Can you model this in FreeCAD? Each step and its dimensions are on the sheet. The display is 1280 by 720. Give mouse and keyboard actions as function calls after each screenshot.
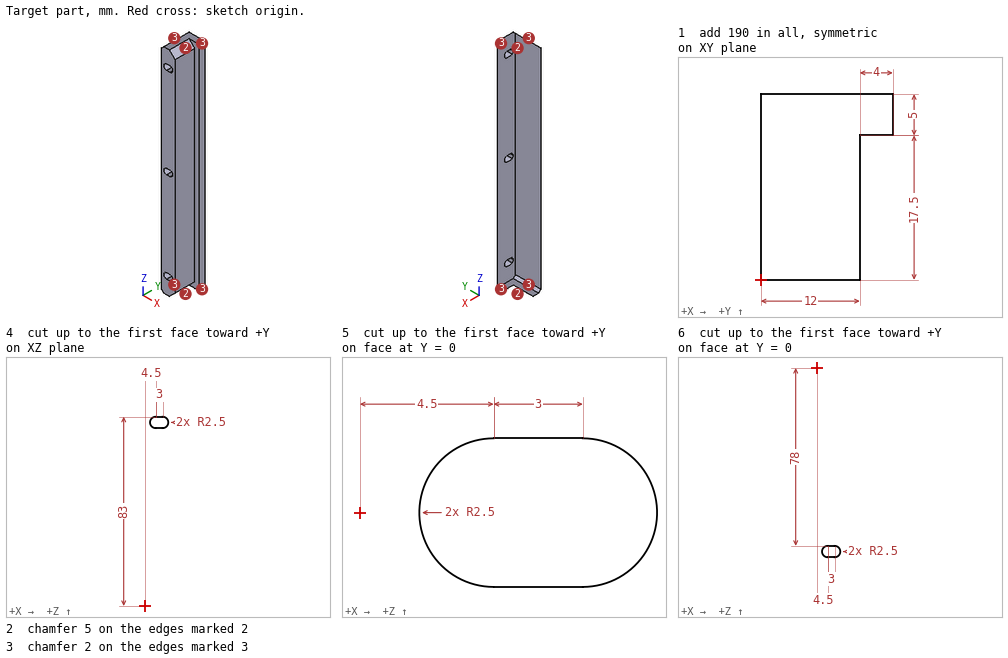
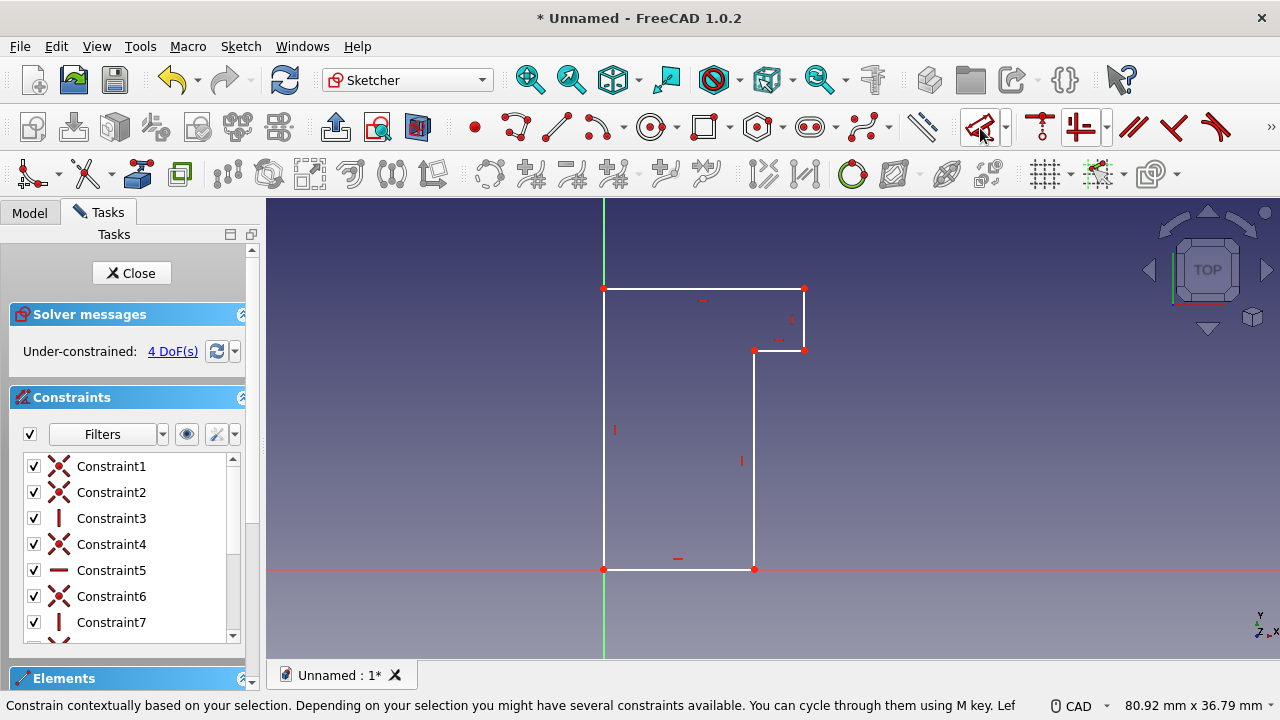
click(769, 351)
click(779, 317)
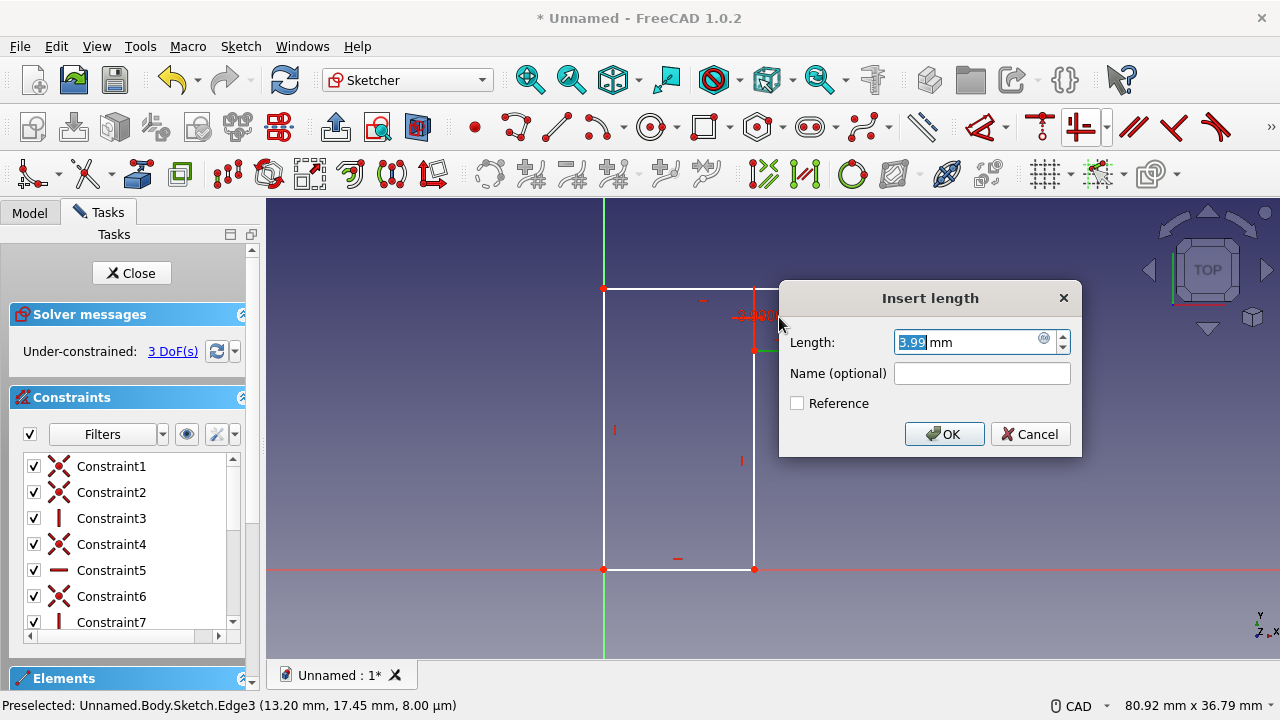
text(4)
key(Return)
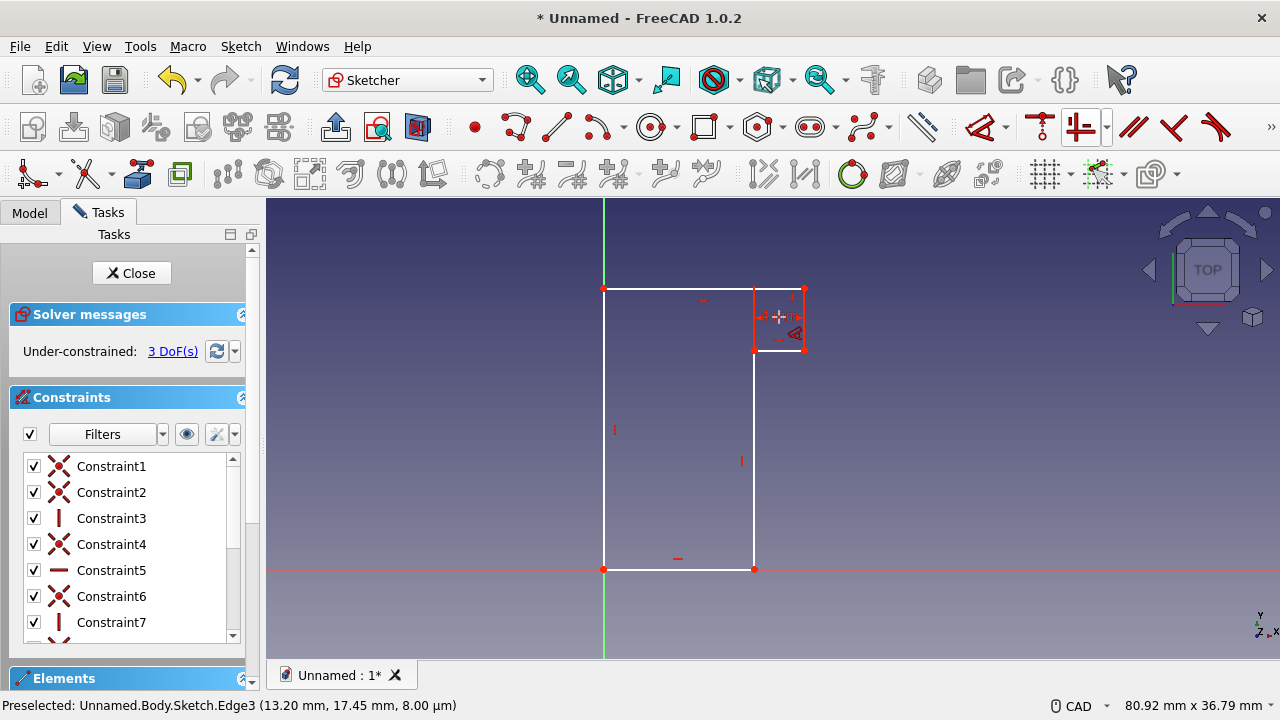
click(804, 332)
click(838, 342)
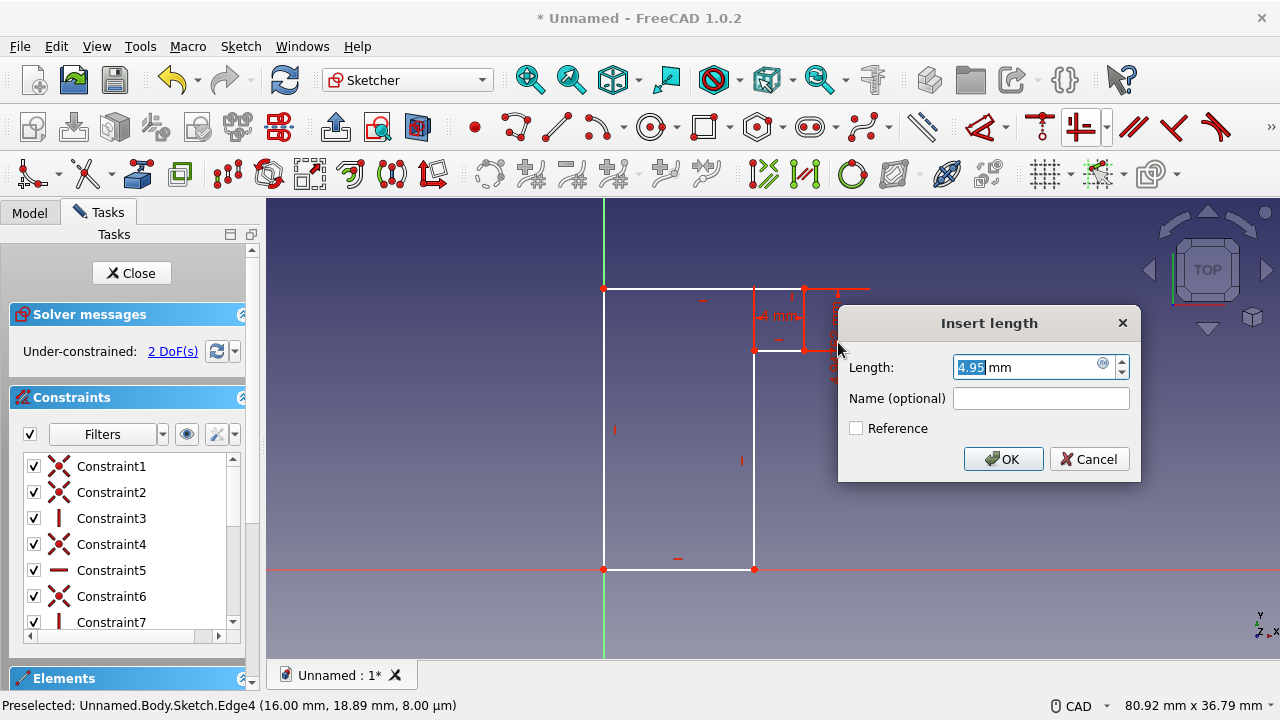
text(5)
key(Return)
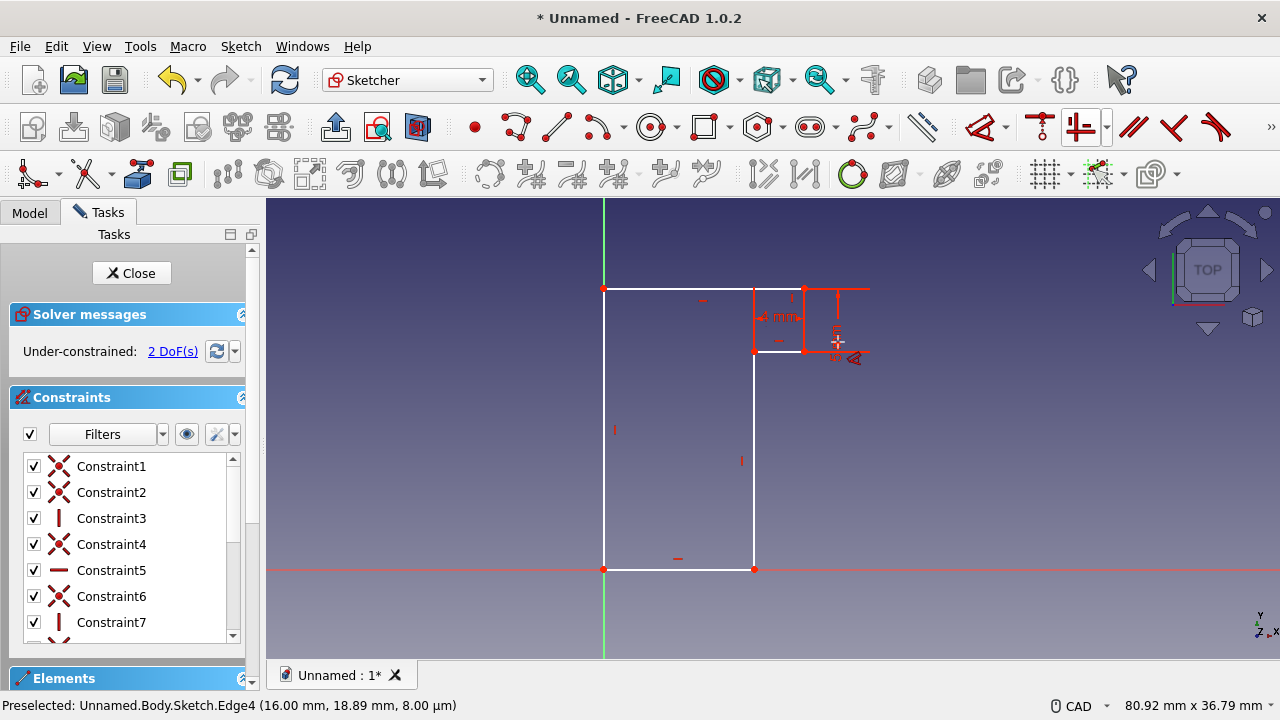
click(649, 570)
click(679, 604)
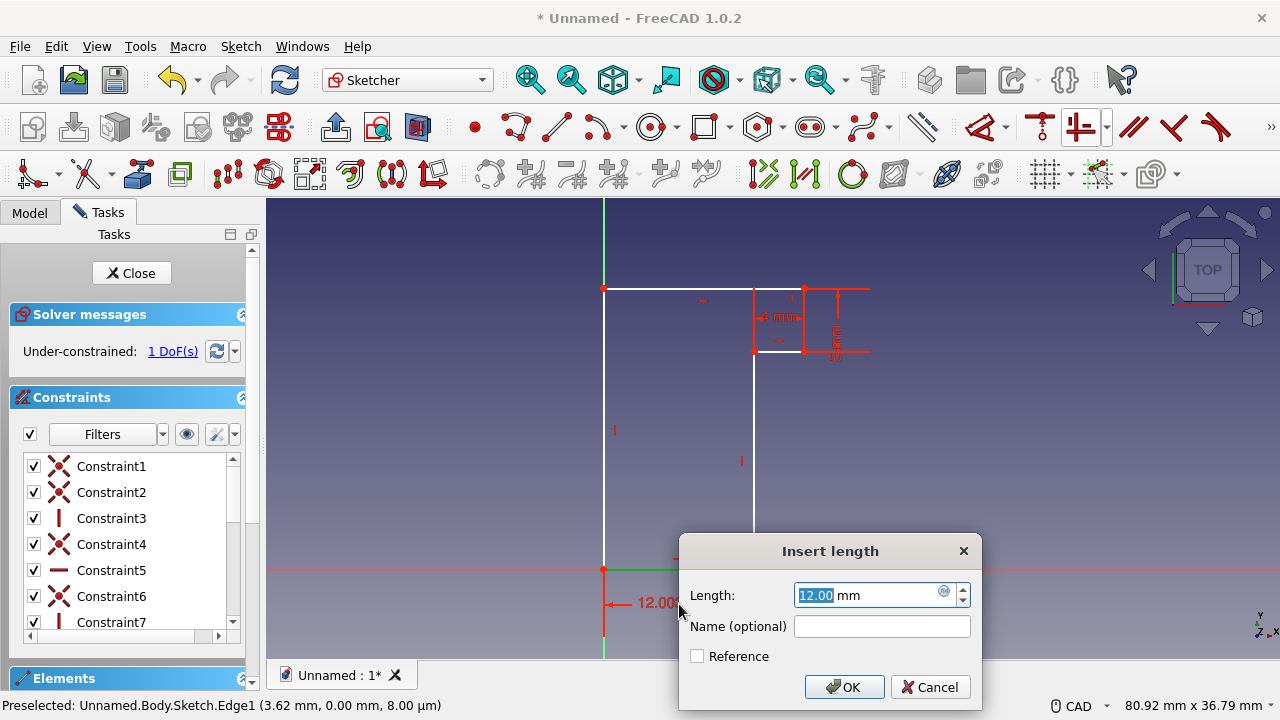
text(12)
key(Return)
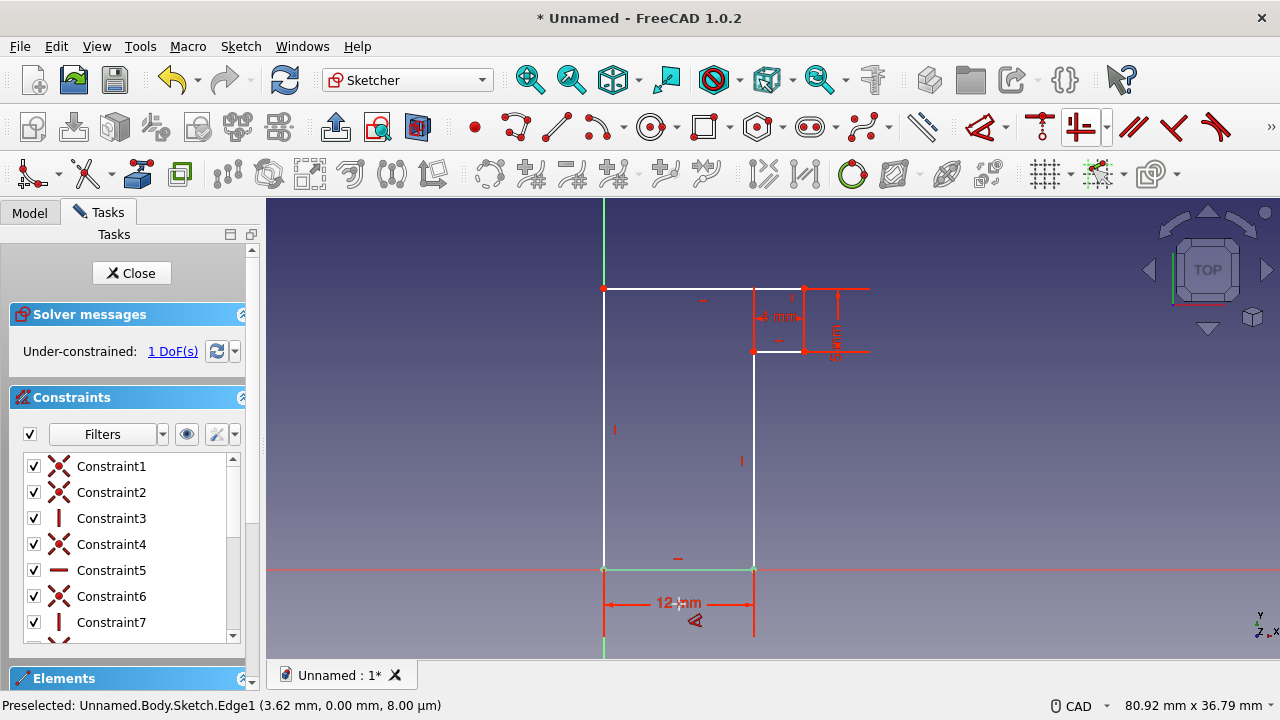
click(754, 504)
click(788, 461)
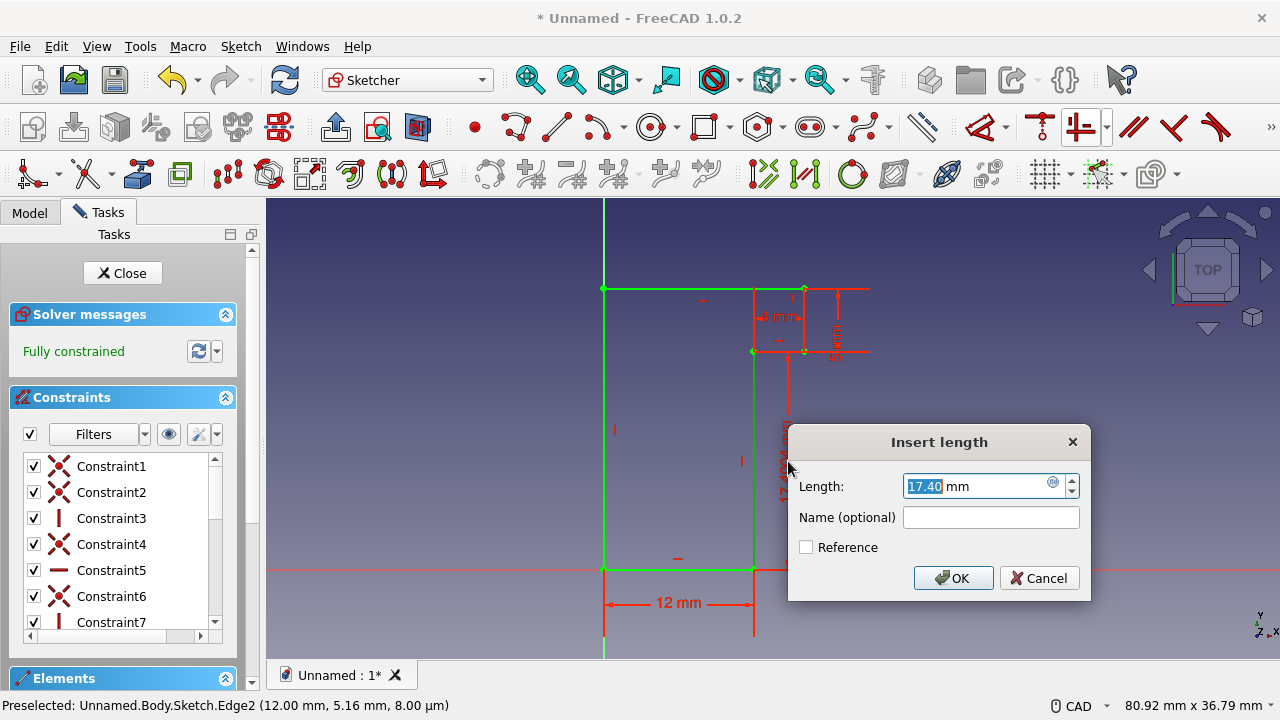
text(17.5)
key(Return)
key(Escape)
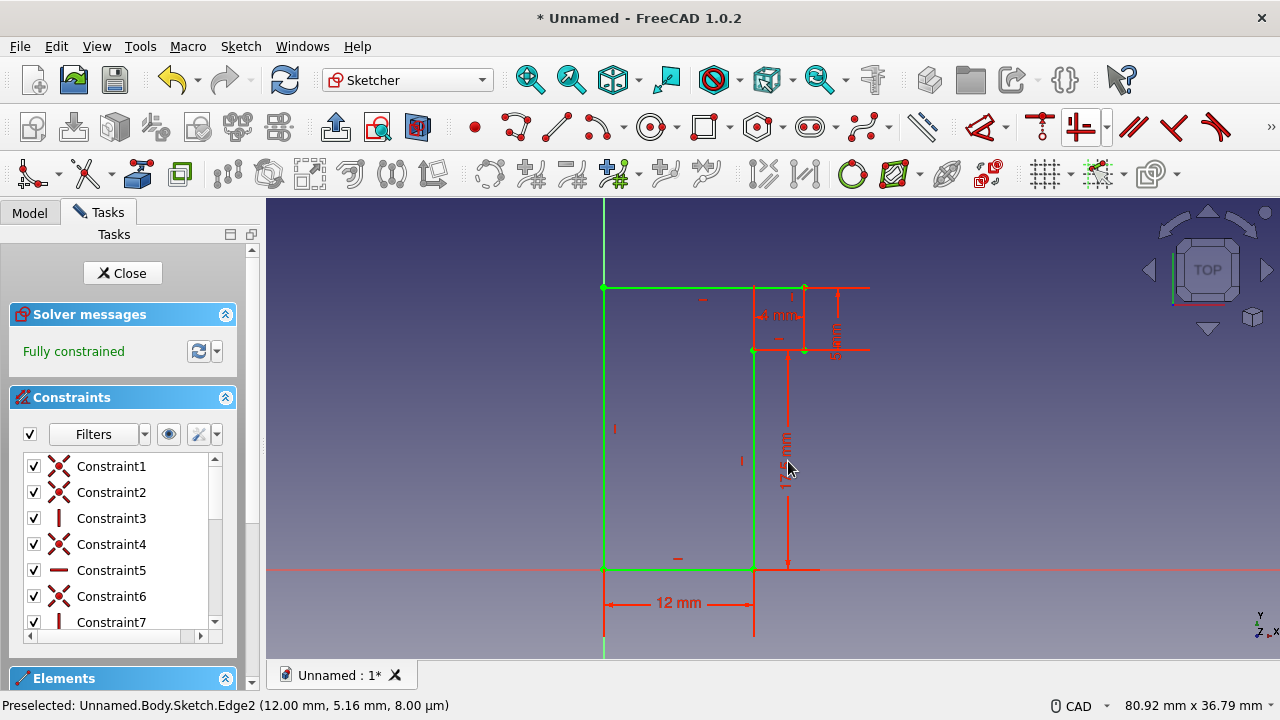
click(123, 273)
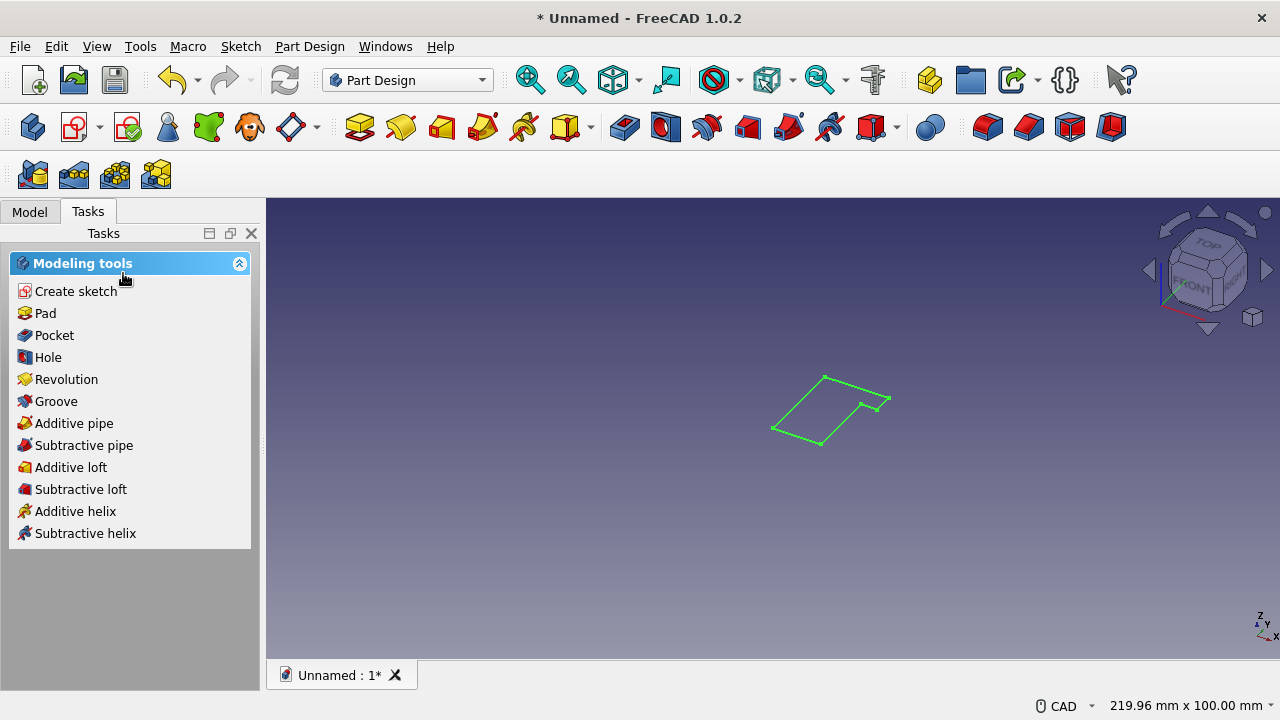
click(360, 128)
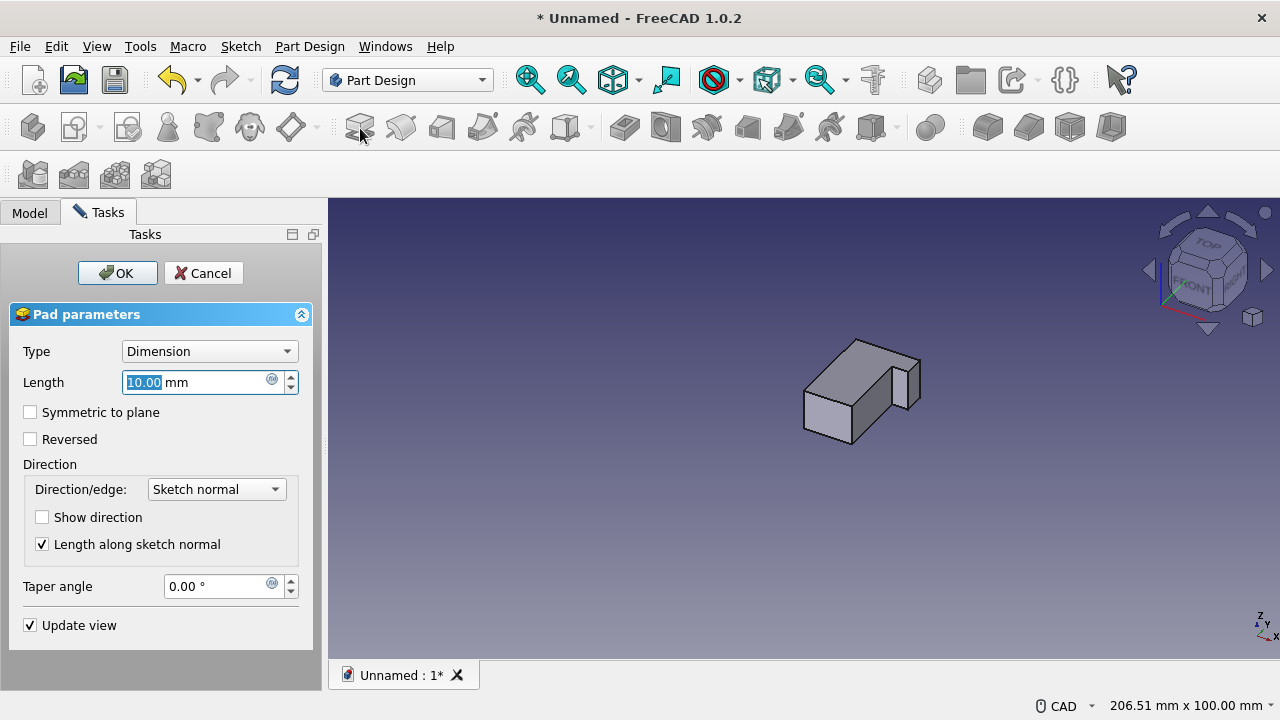
text(190)
key(Tab)